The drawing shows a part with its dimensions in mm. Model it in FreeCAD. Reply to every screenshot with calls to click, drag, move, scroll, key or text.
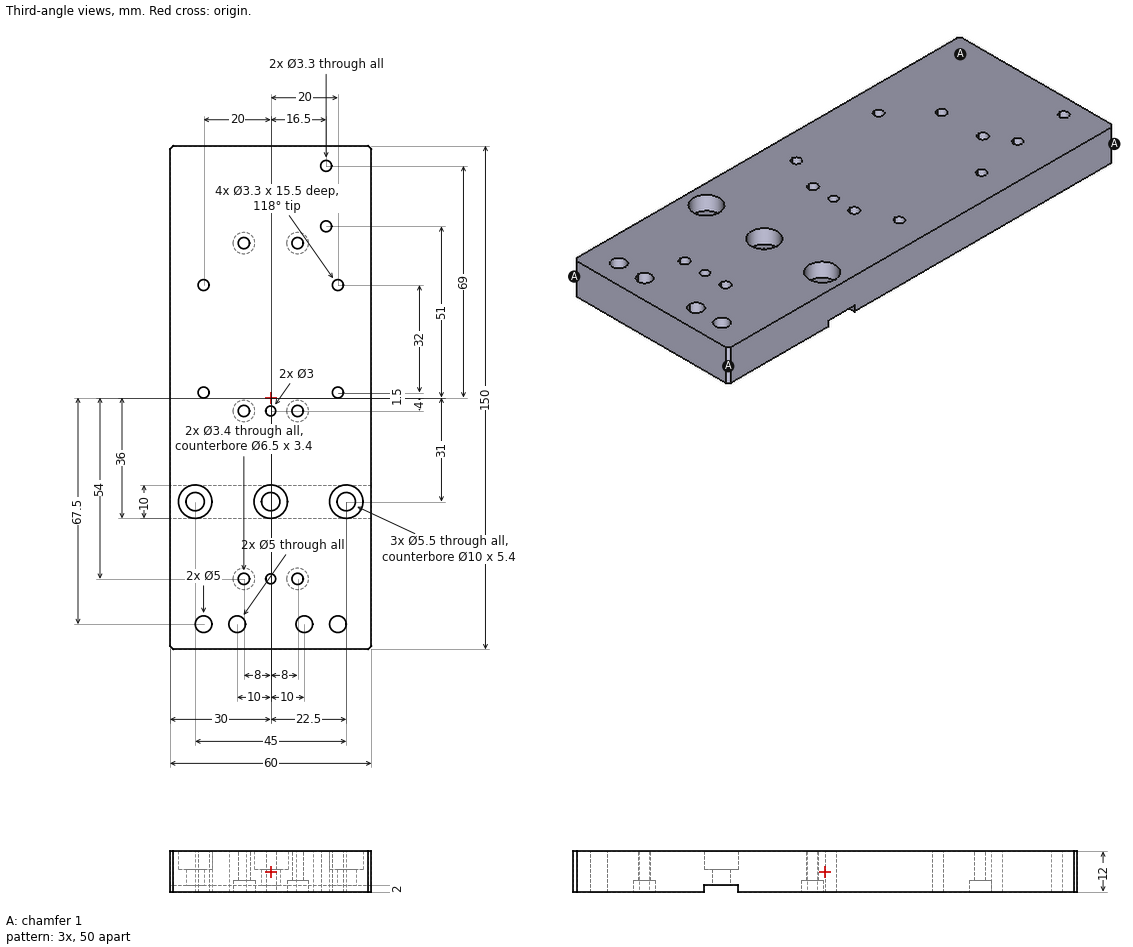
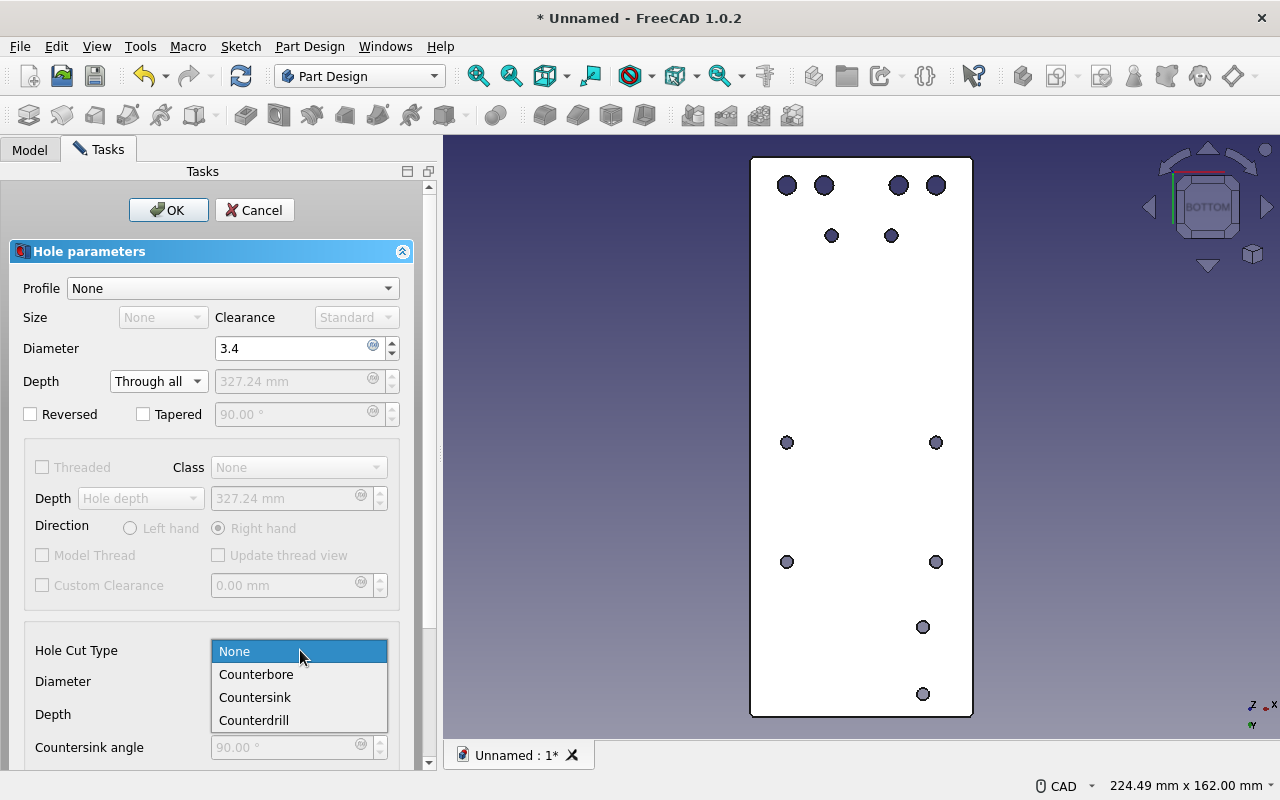
click(298, 674)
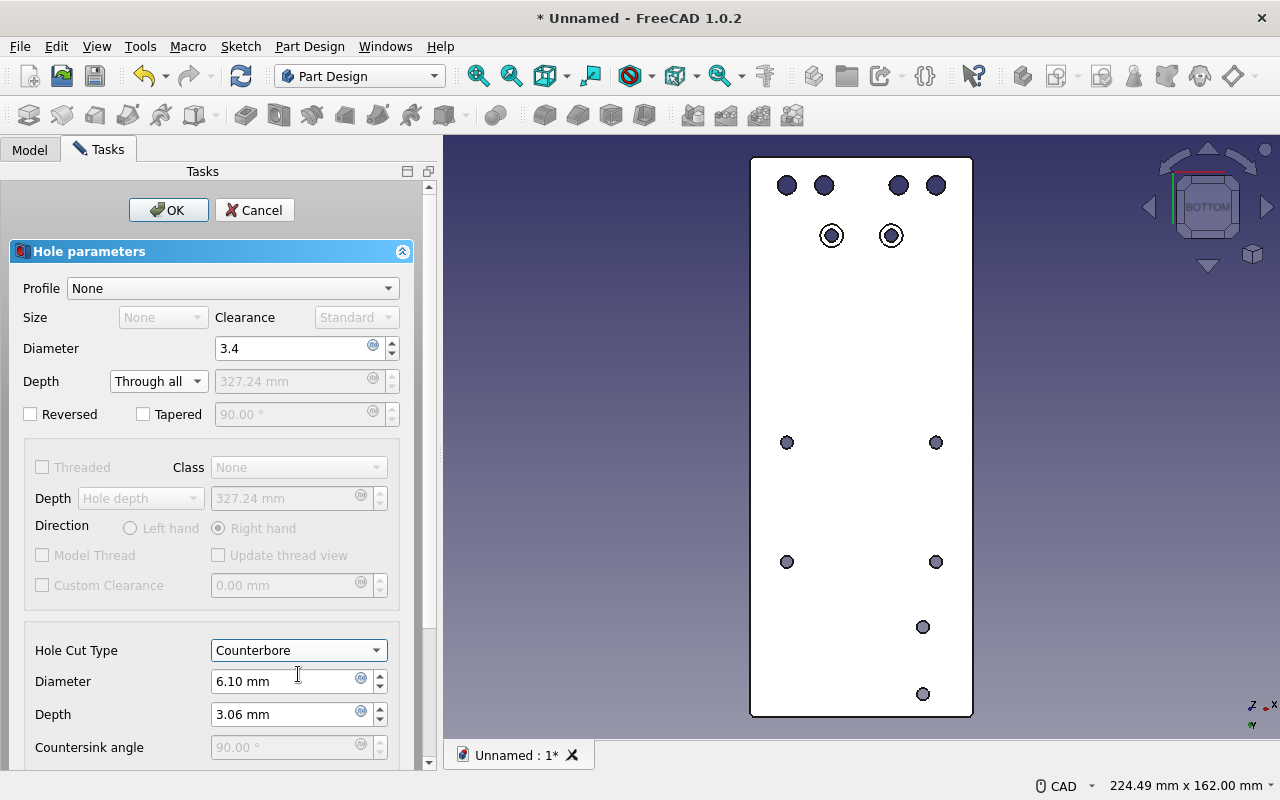
triple_click(292, 682)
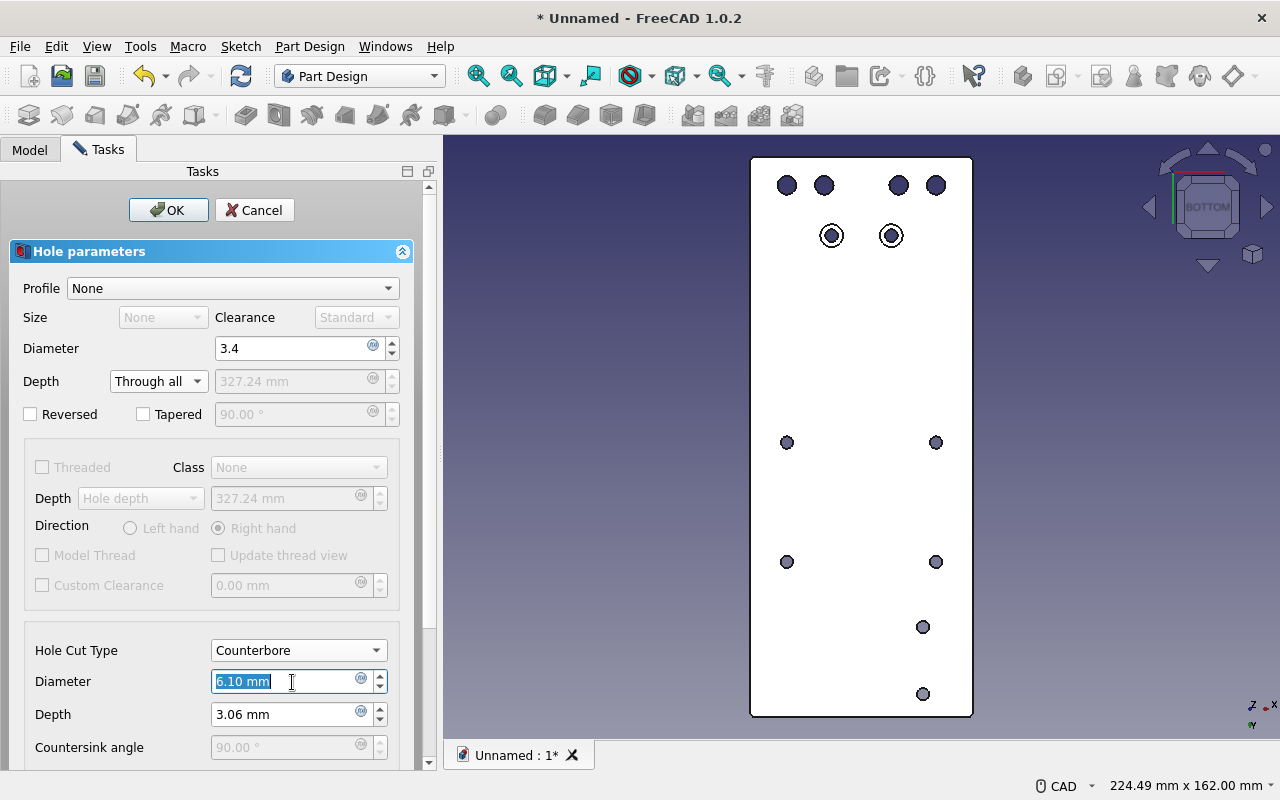
text(6.5)
key(Tab)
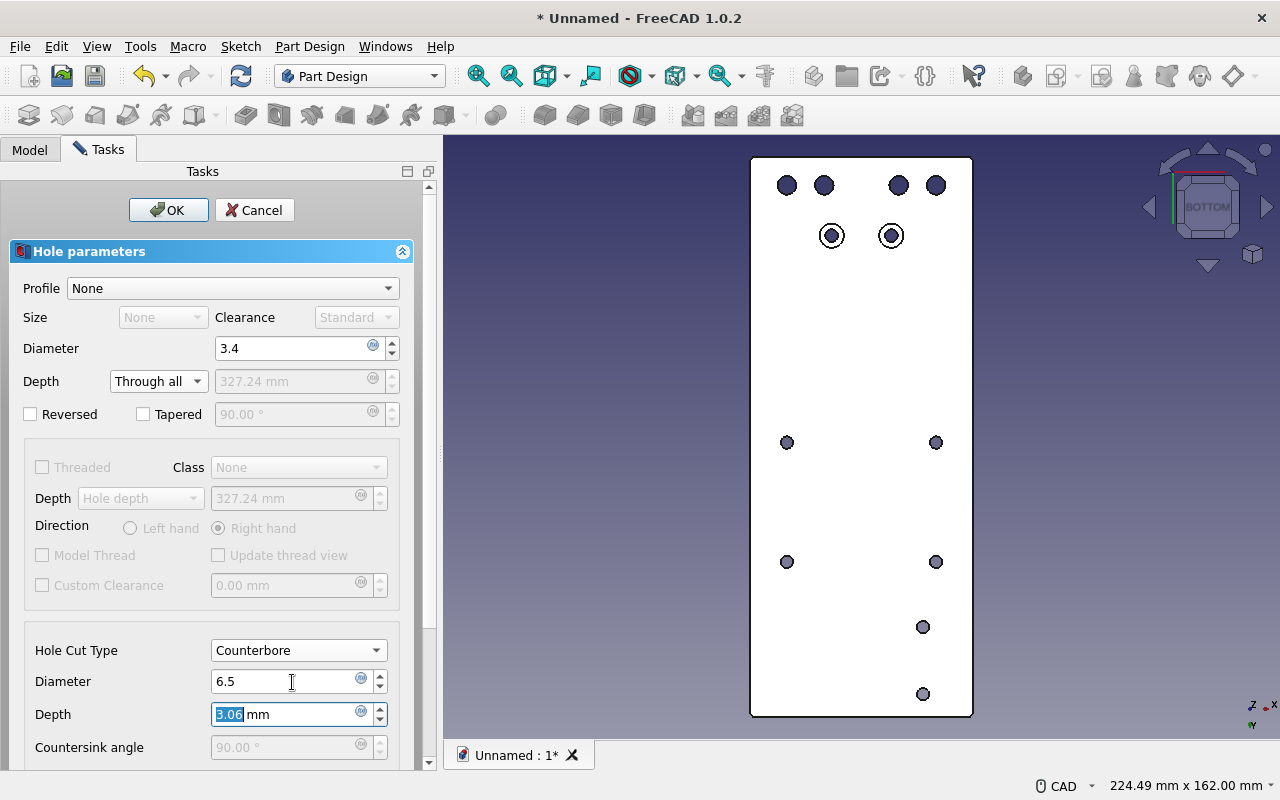
text(3.4)
key(Tab)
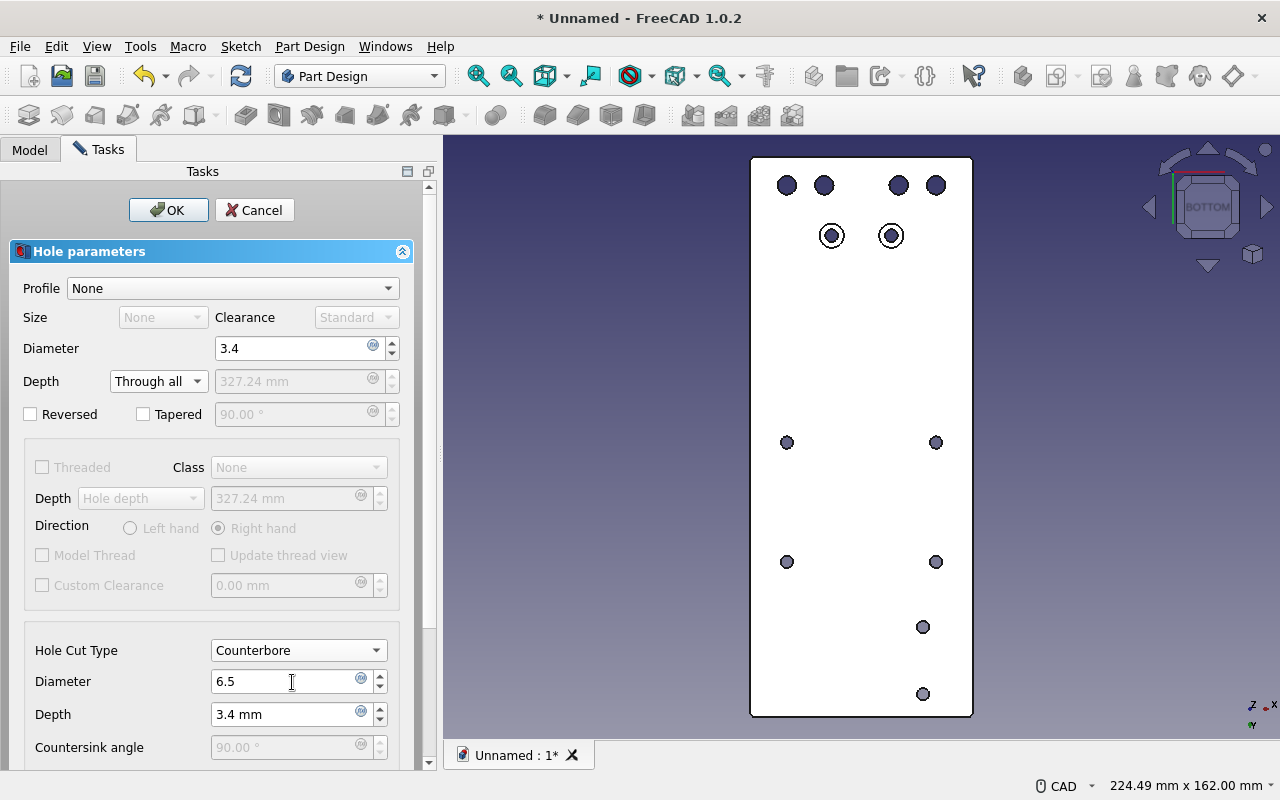
click(169, 210)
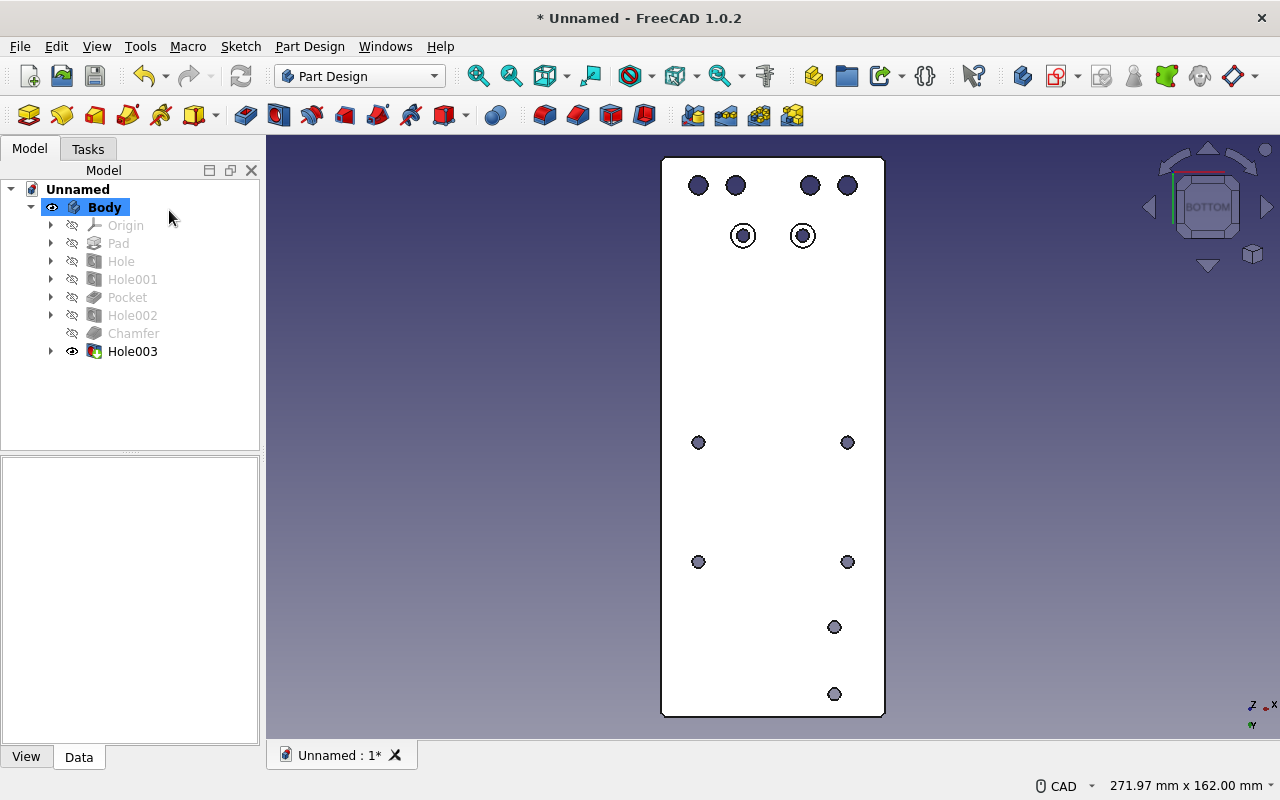
click(117, 351)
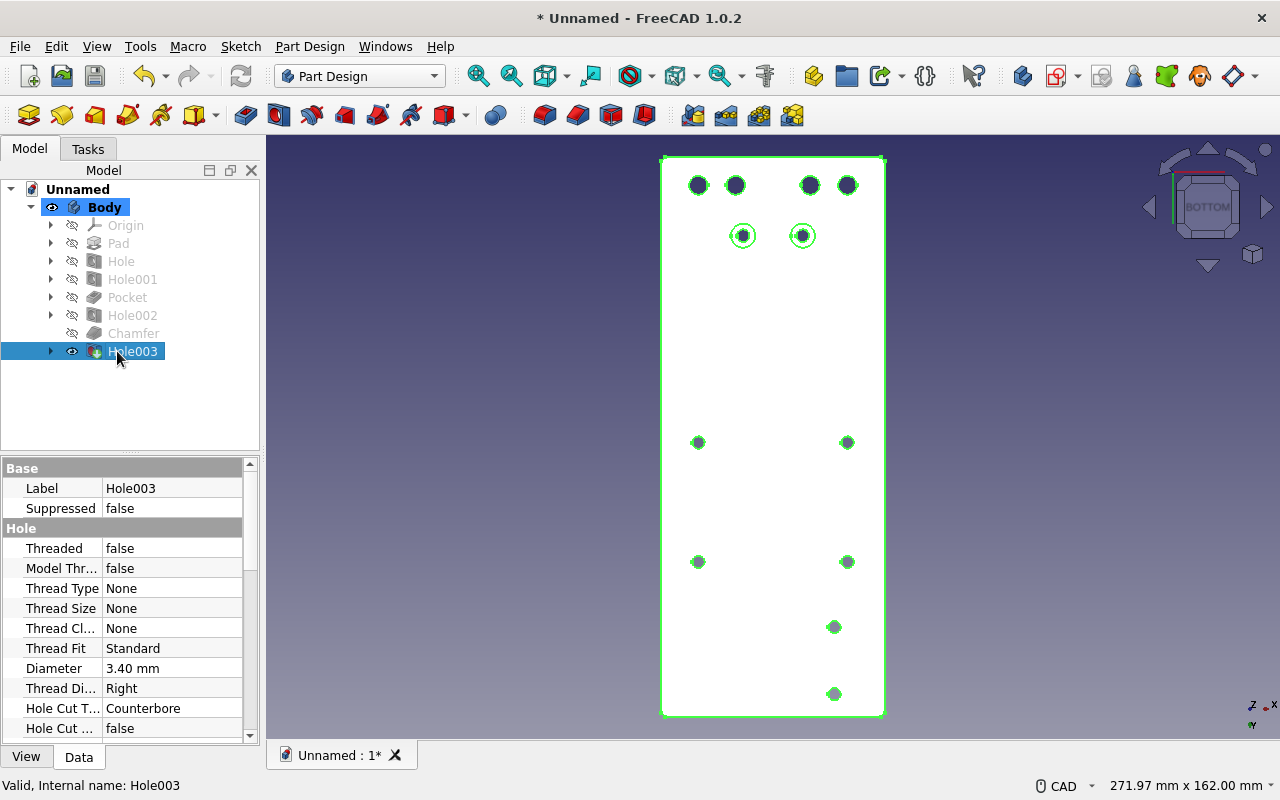
click(726, 116)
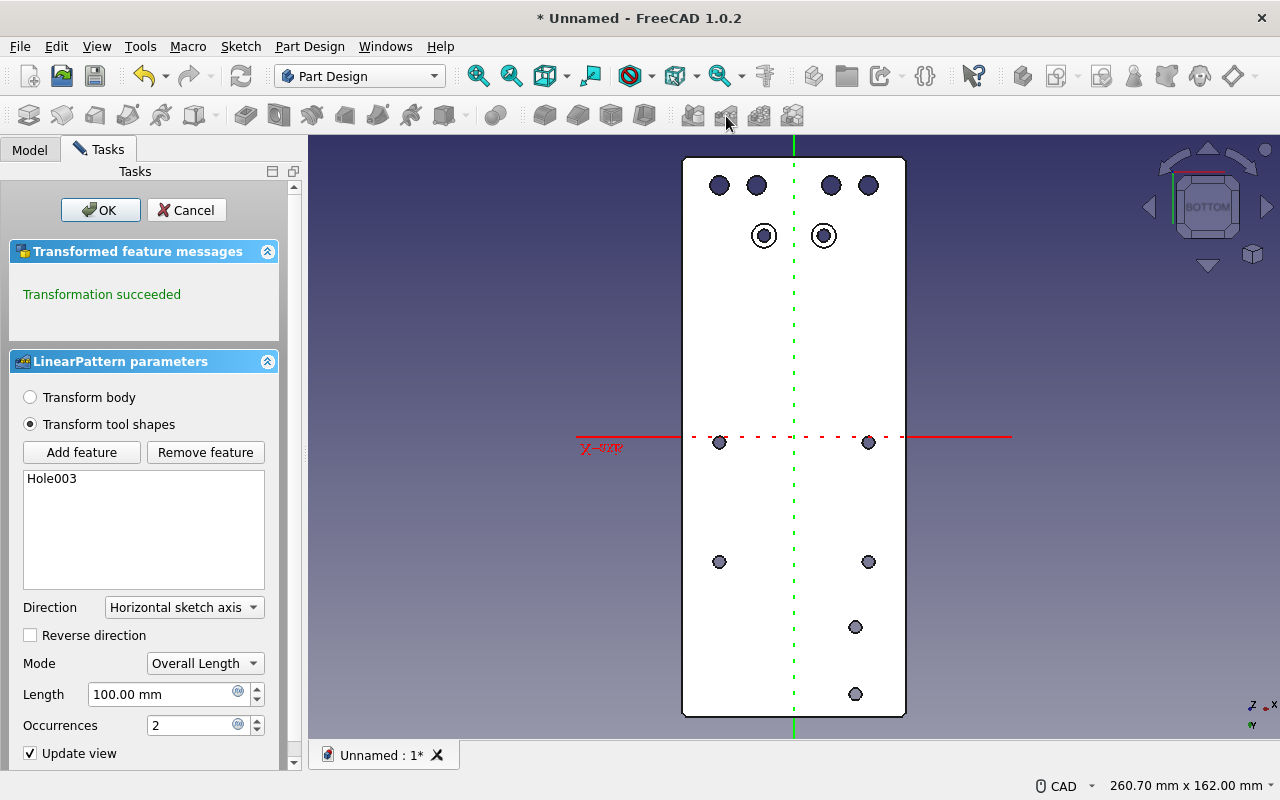
click(185, 608)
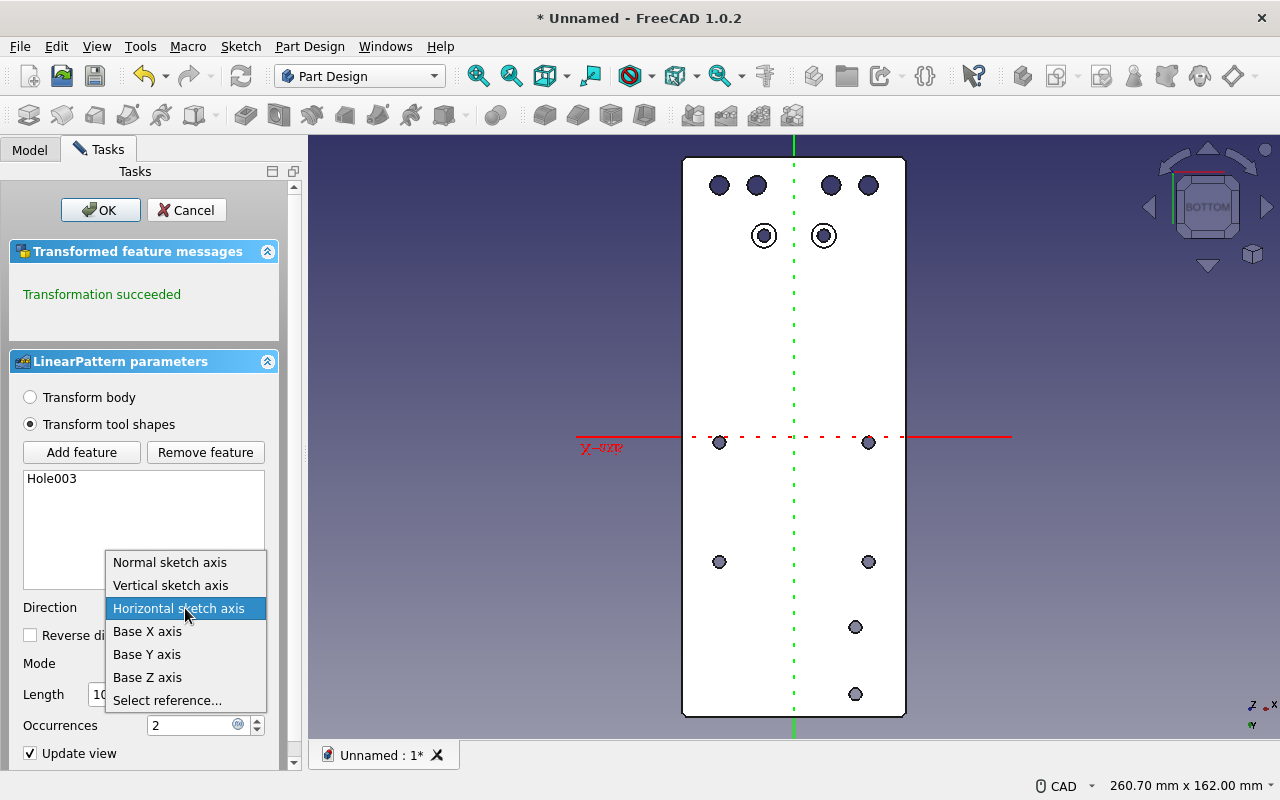
click(184, 654)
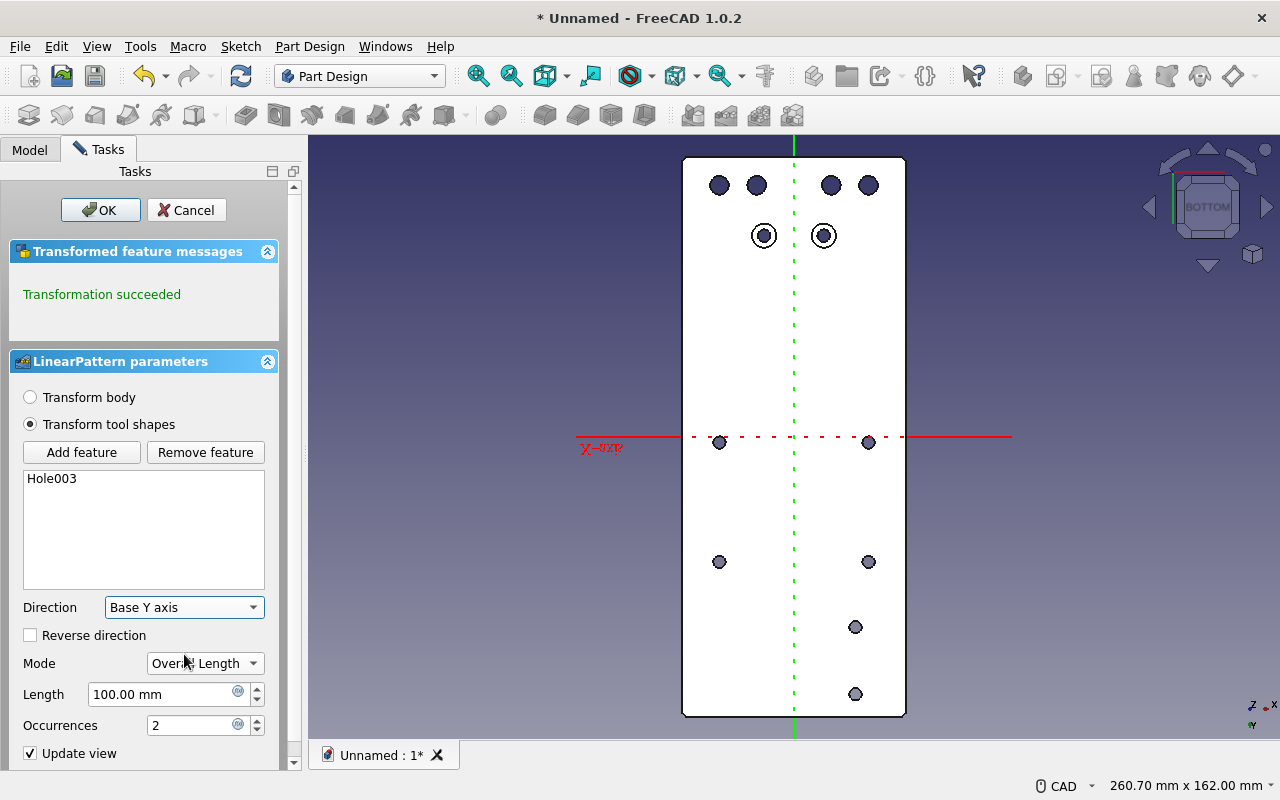
click(206, 664)